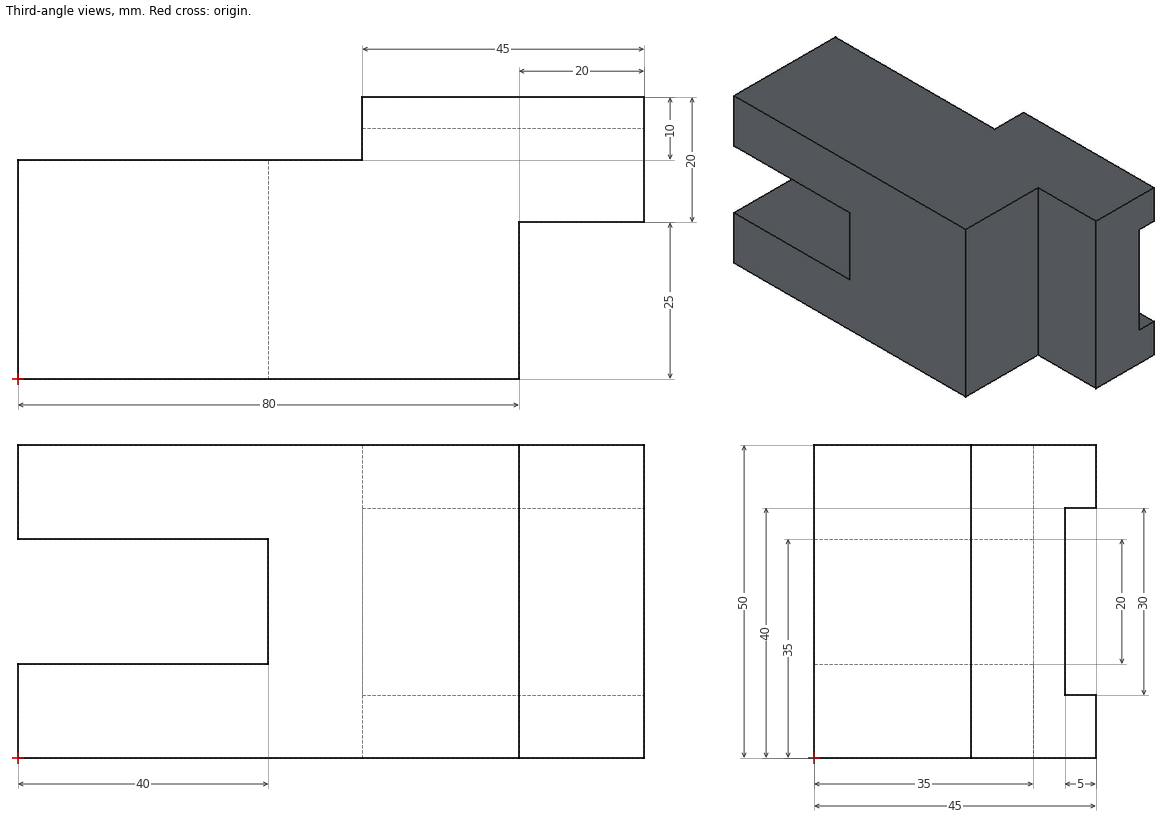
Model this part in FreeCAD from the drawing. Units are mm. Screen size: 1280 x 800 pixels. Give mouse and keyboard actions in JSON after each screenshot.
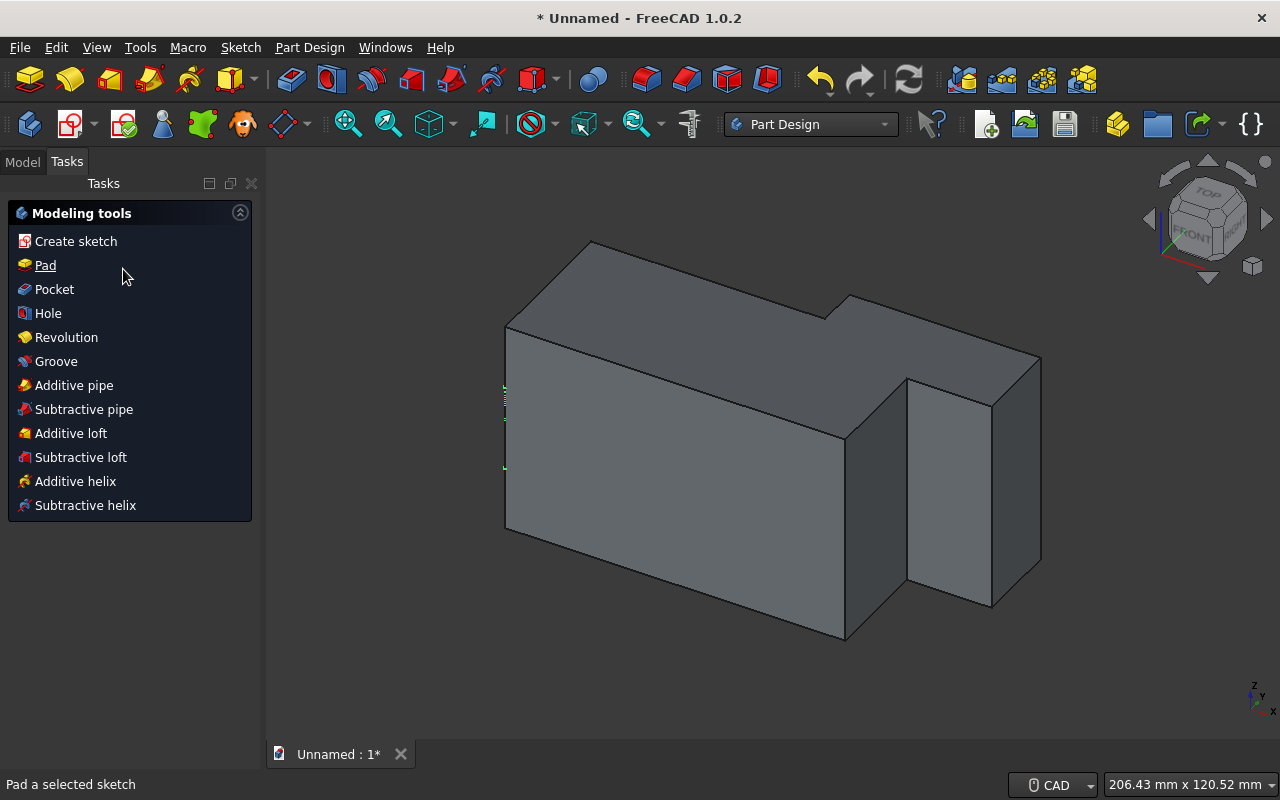
{"action": "left_click", "coordinate": [292, 80]}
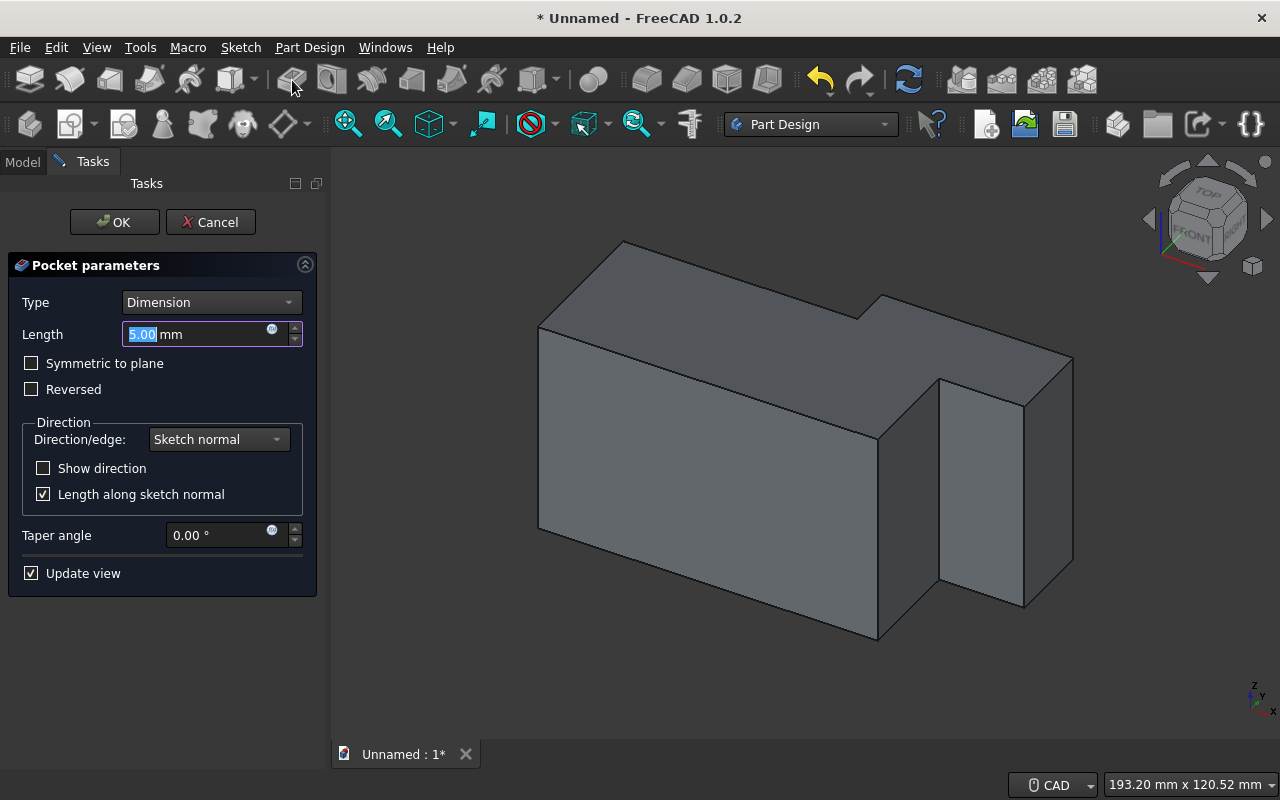
{"action": "type", "text": "40"}
{"action": "key", "text": "Tab"}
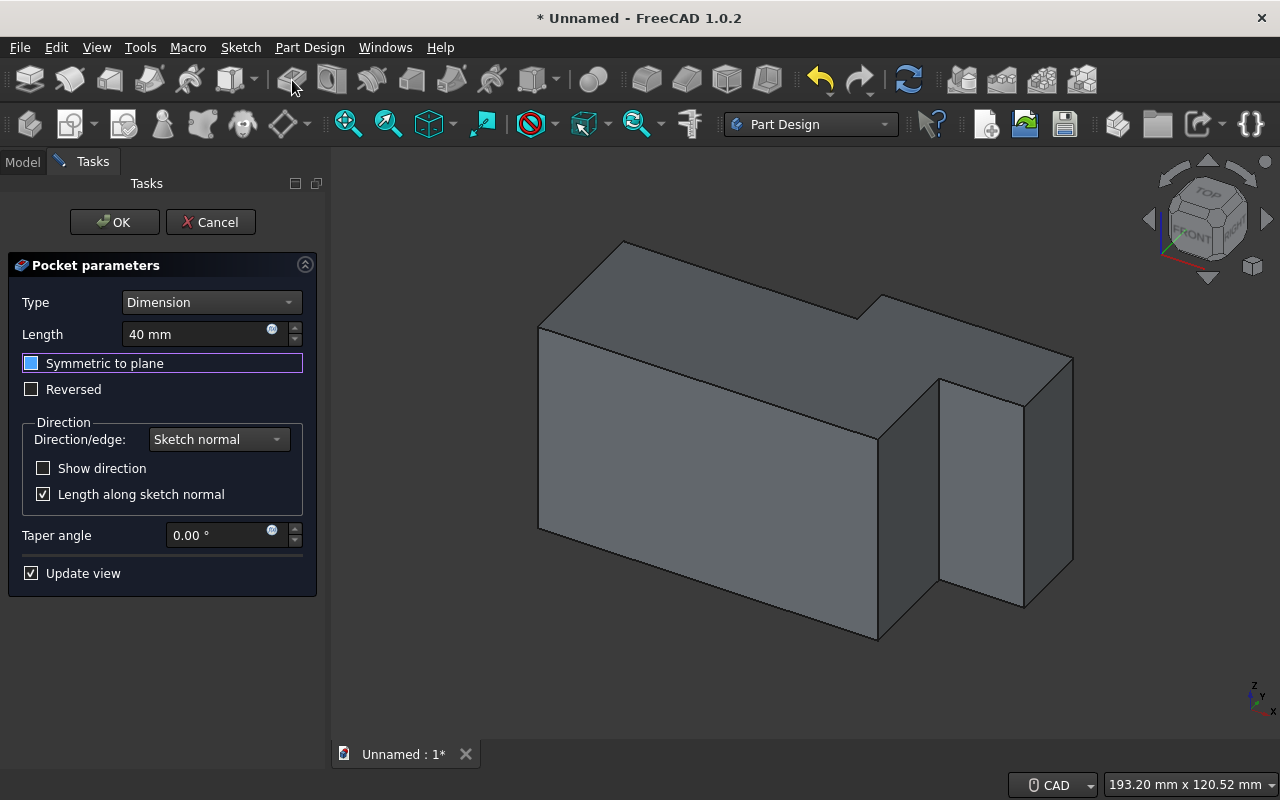
{"action": "left_click", "coordinate": [30, 389]}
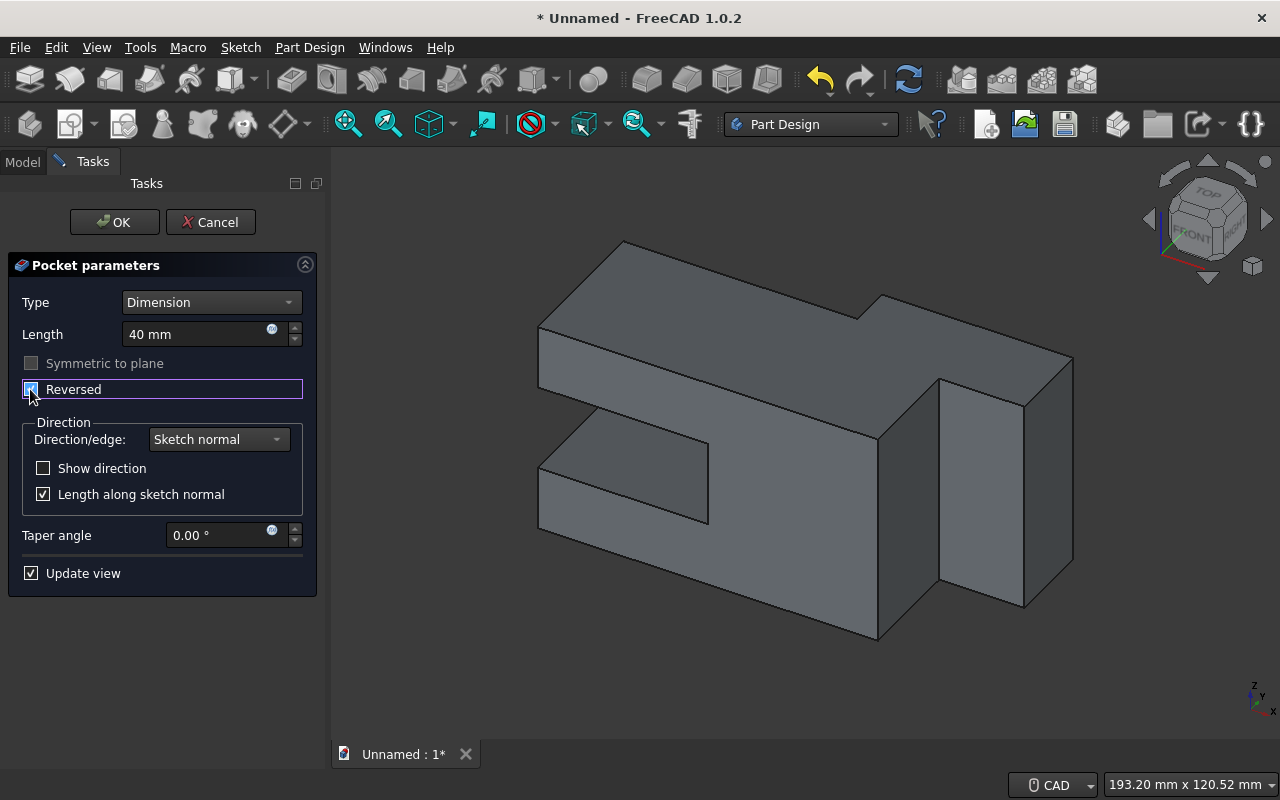
{"action": "left_click", "coordinate": [115, 222]}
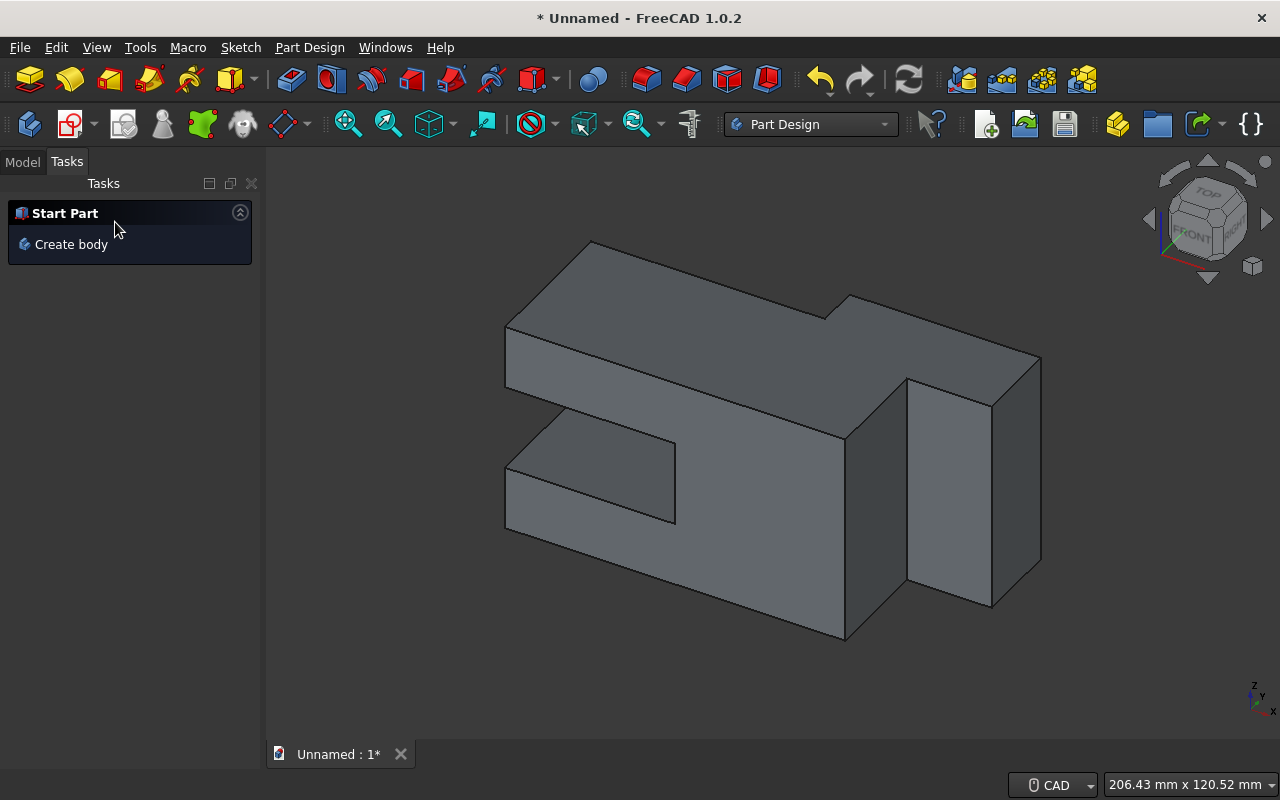
{"action": "key", "text": "6"}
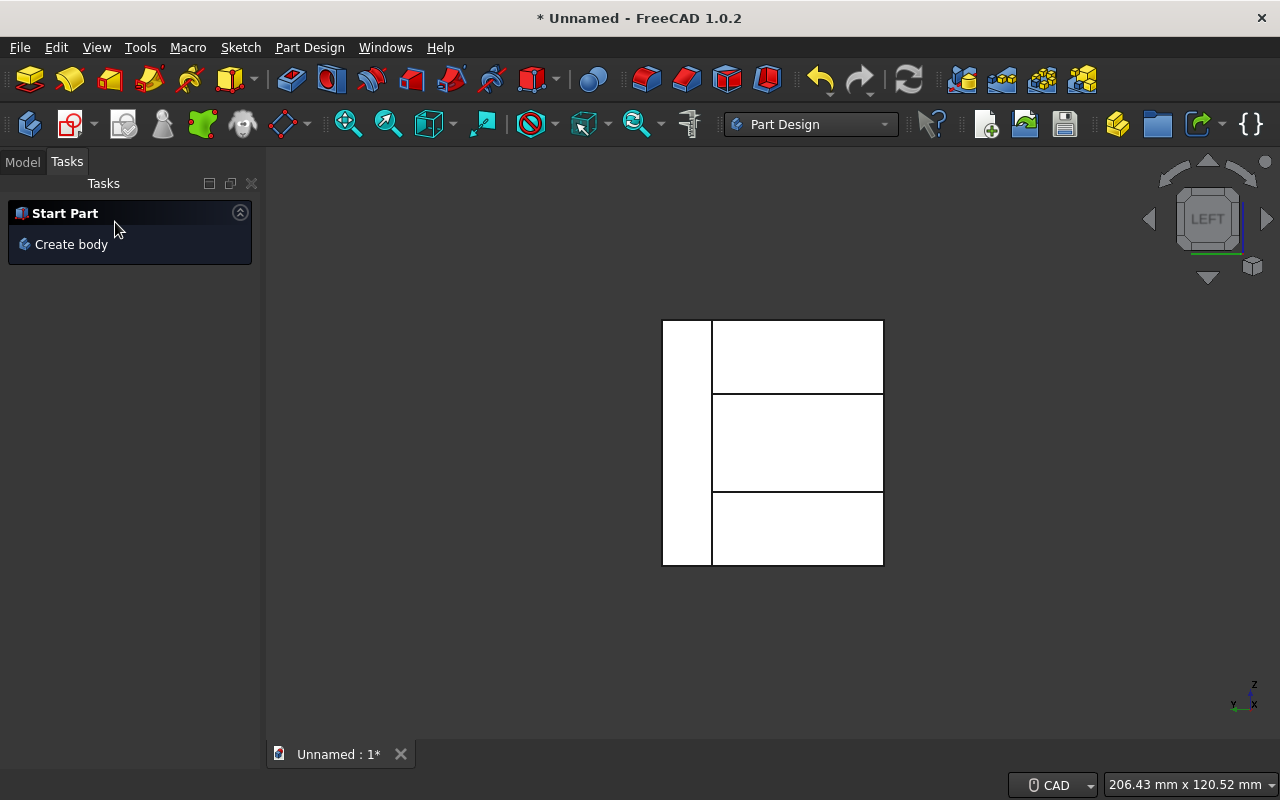
{"action": "left_click", "coordinate": [350, 124]}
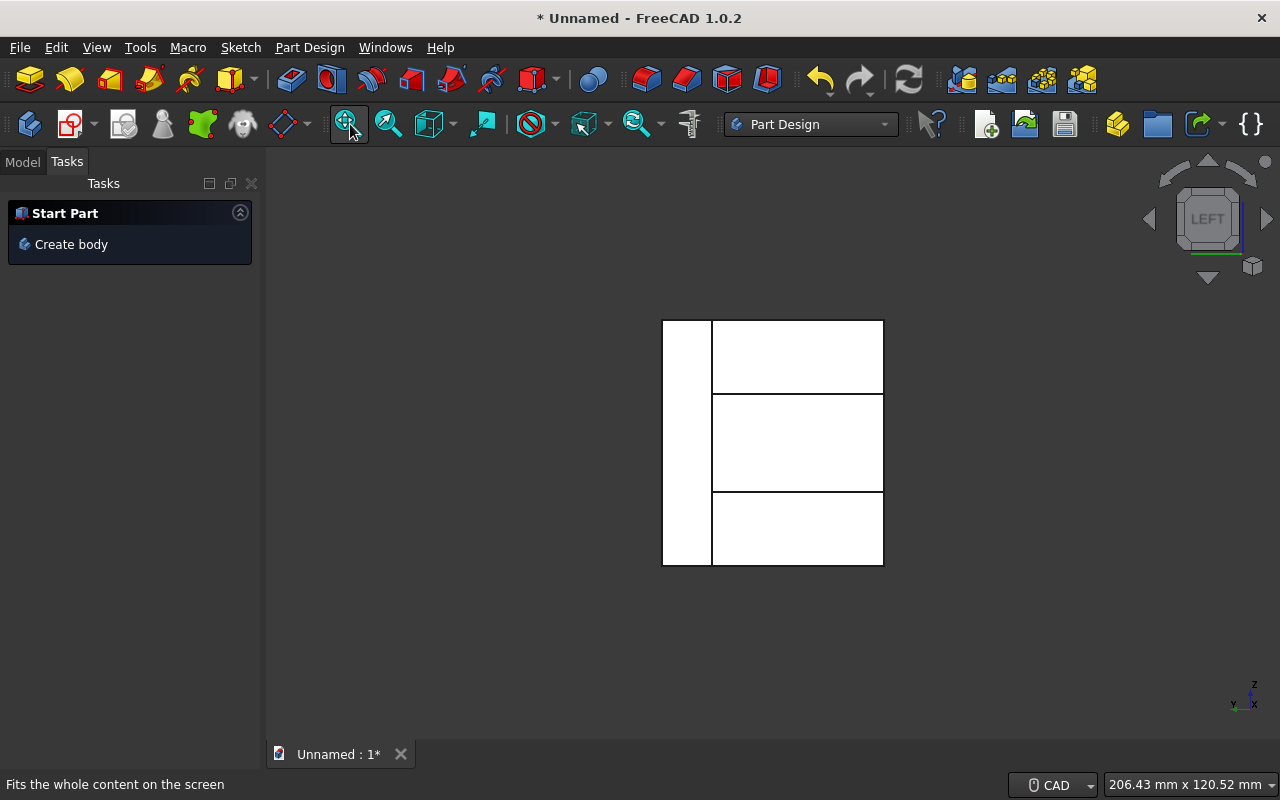
{"action": "left_click", "coordinate": [687, 372]}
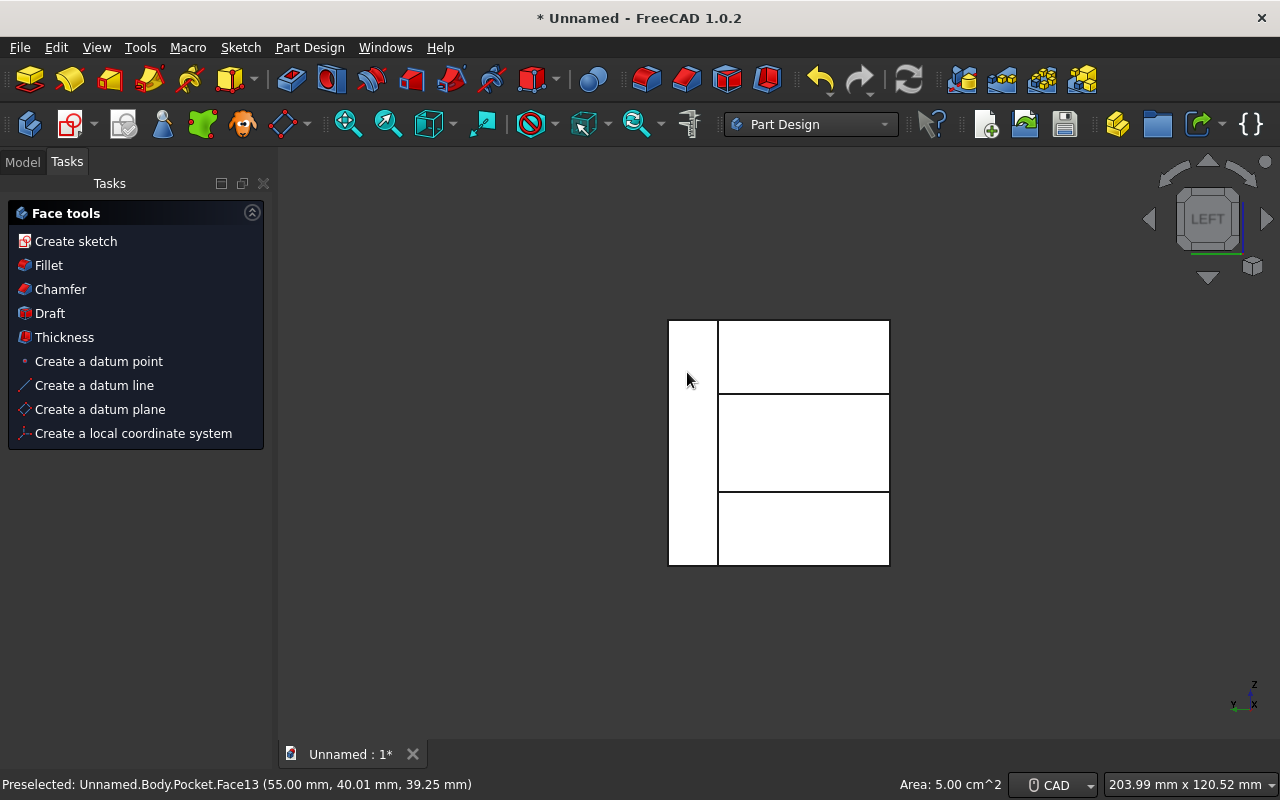
{"action": "left_click", "coordinate": [70, 124]}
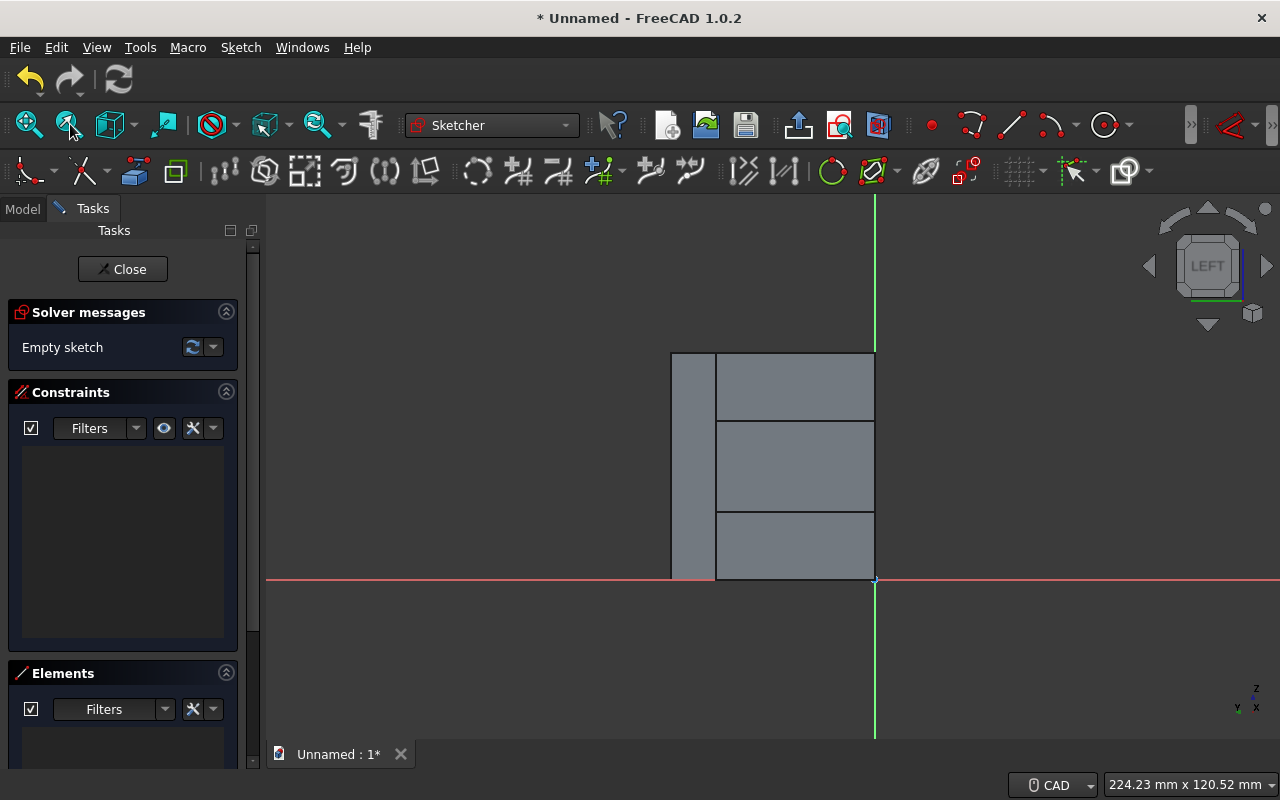
{"action": "left_click", "coordinate": [880, 126]}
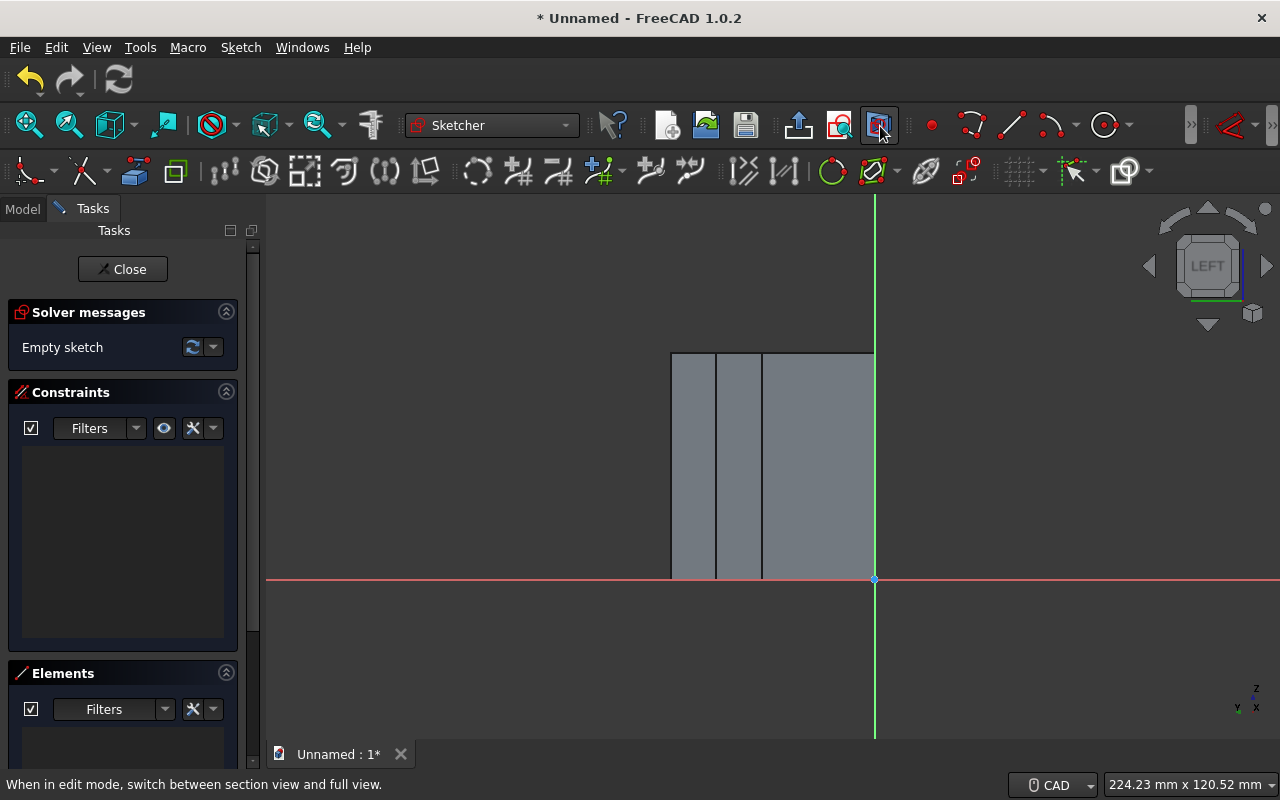
{"action": "scroll", "coordinate": [856, 517], "scroll_direction": "up", "scroll_amount": 3}